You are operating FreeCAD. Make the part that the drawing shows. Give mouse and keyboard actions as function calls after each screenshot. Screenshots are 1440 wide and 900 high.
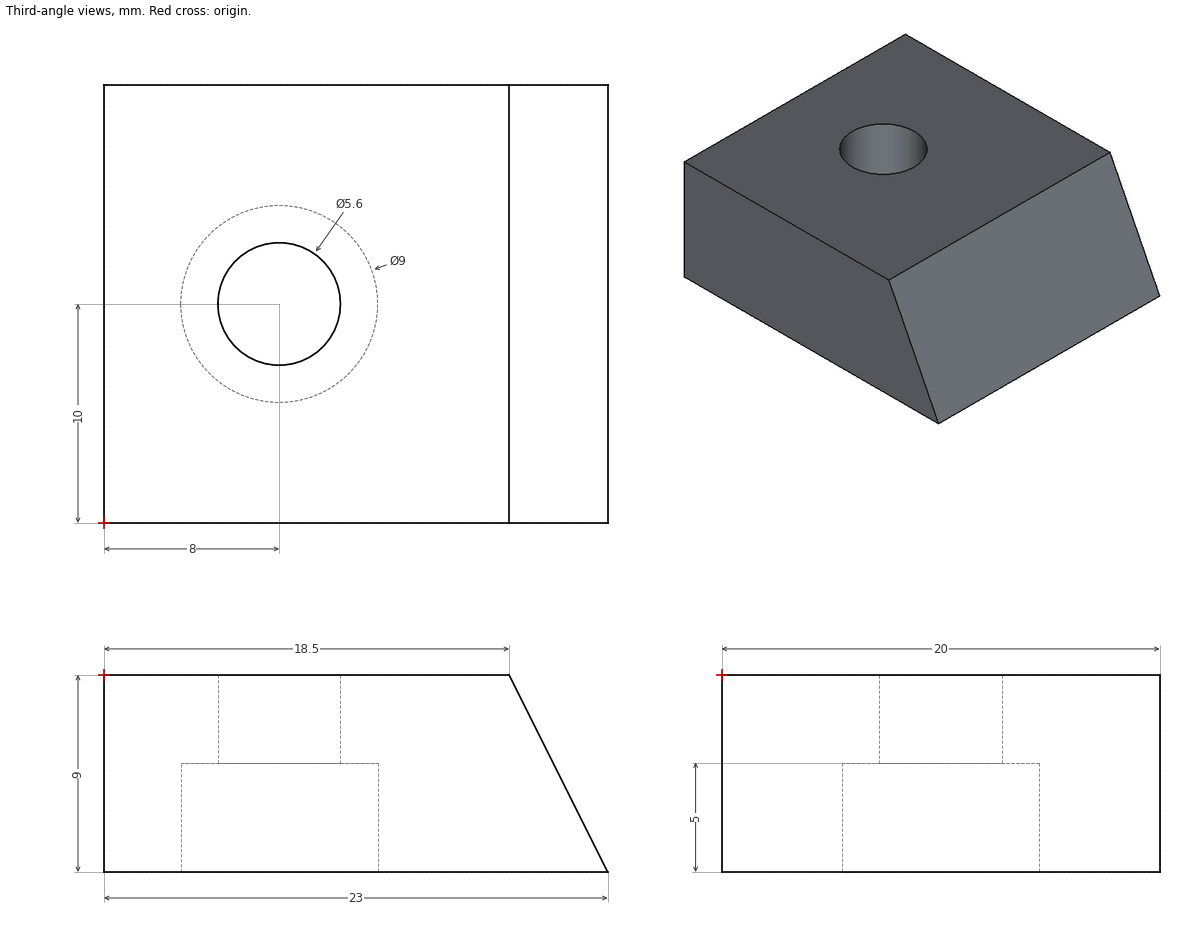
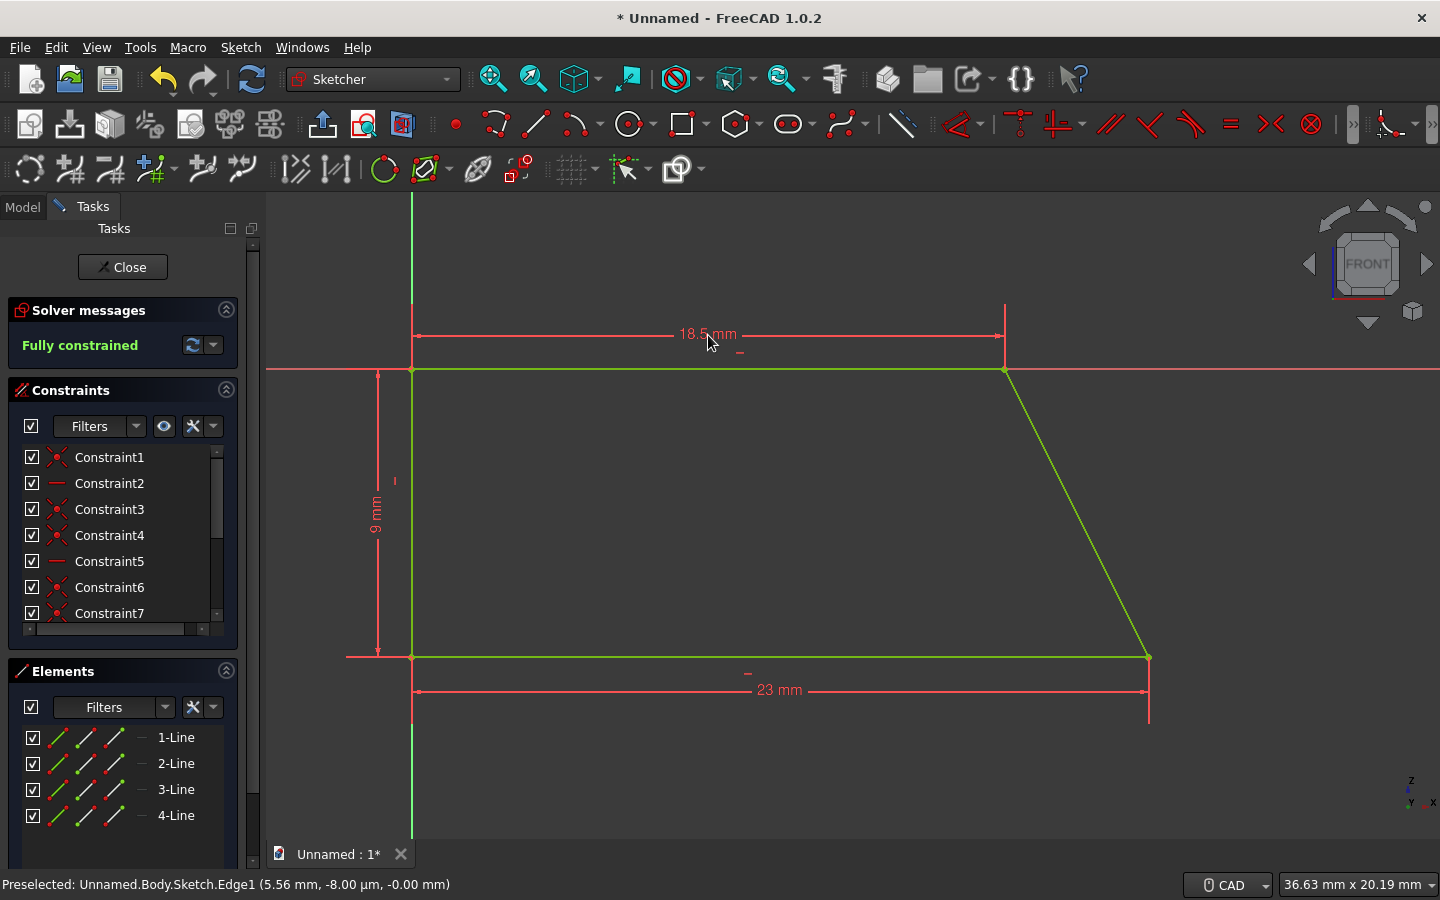
click(123, 267)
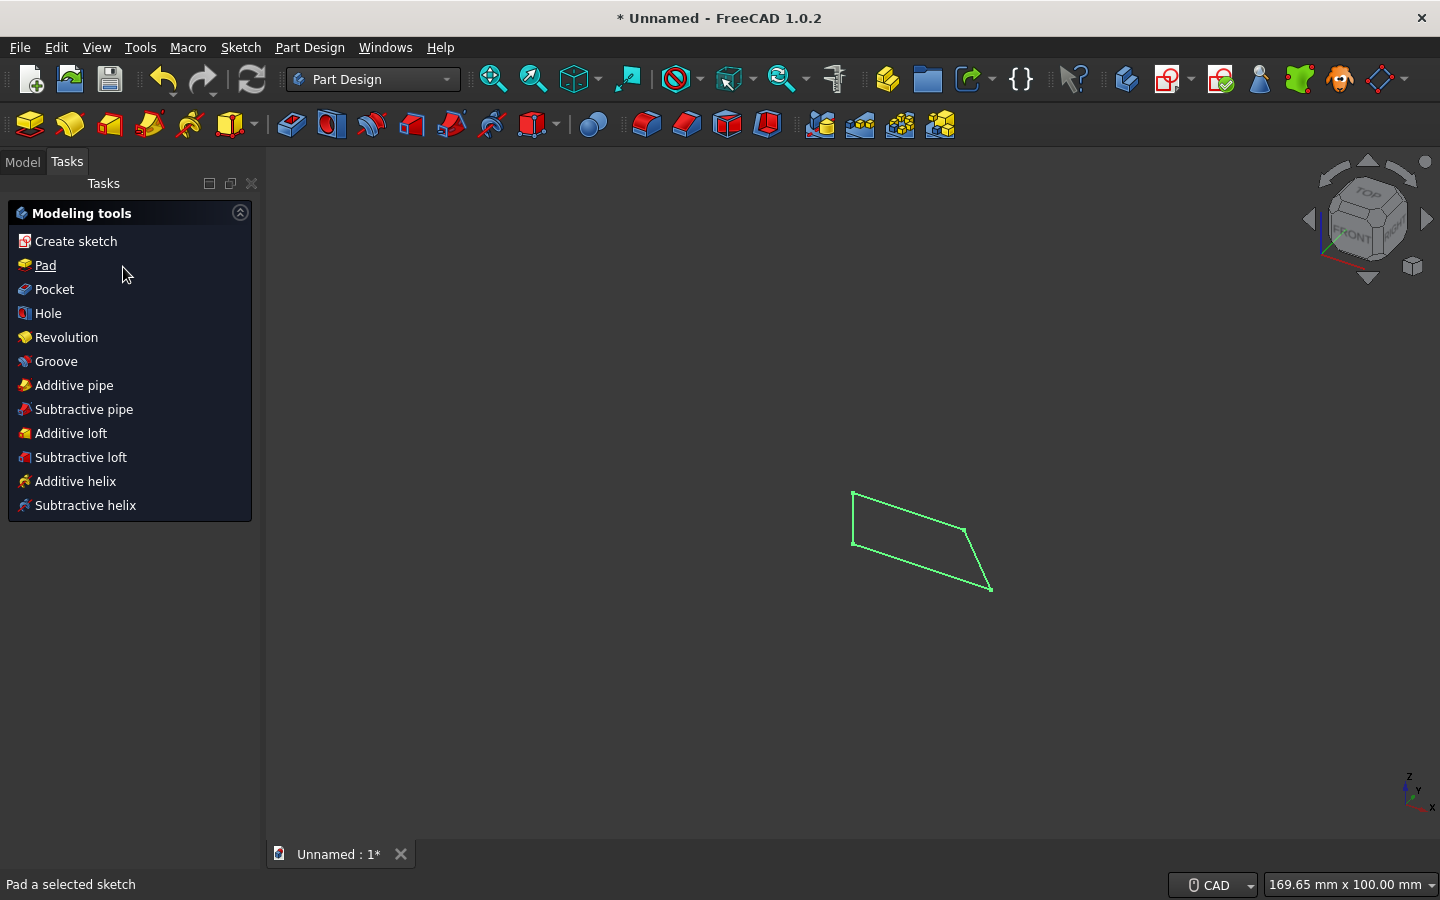
click(30, 124)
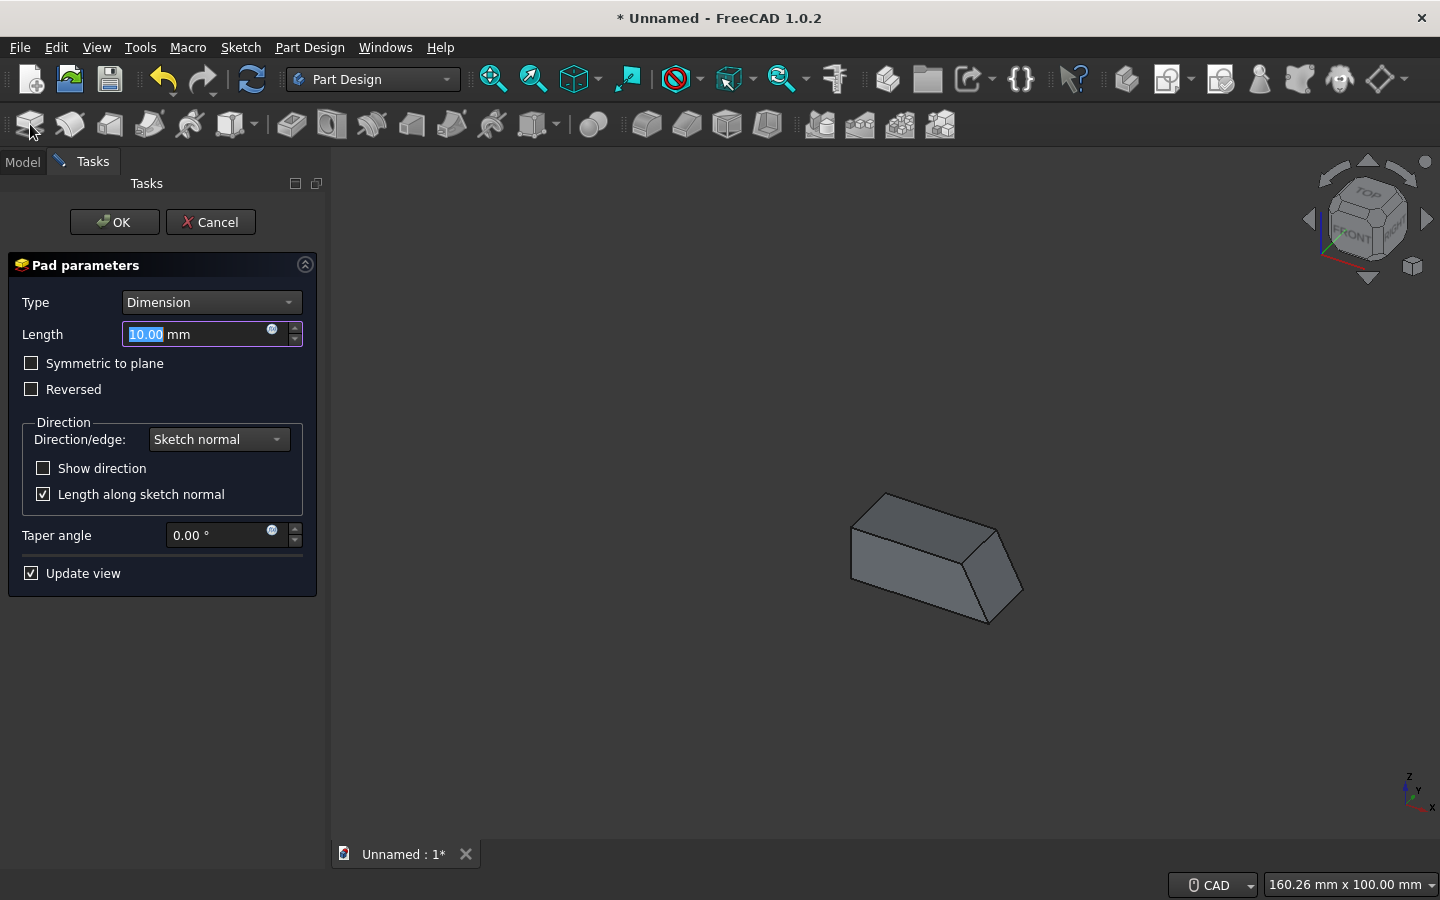
text(20)
key(Tab)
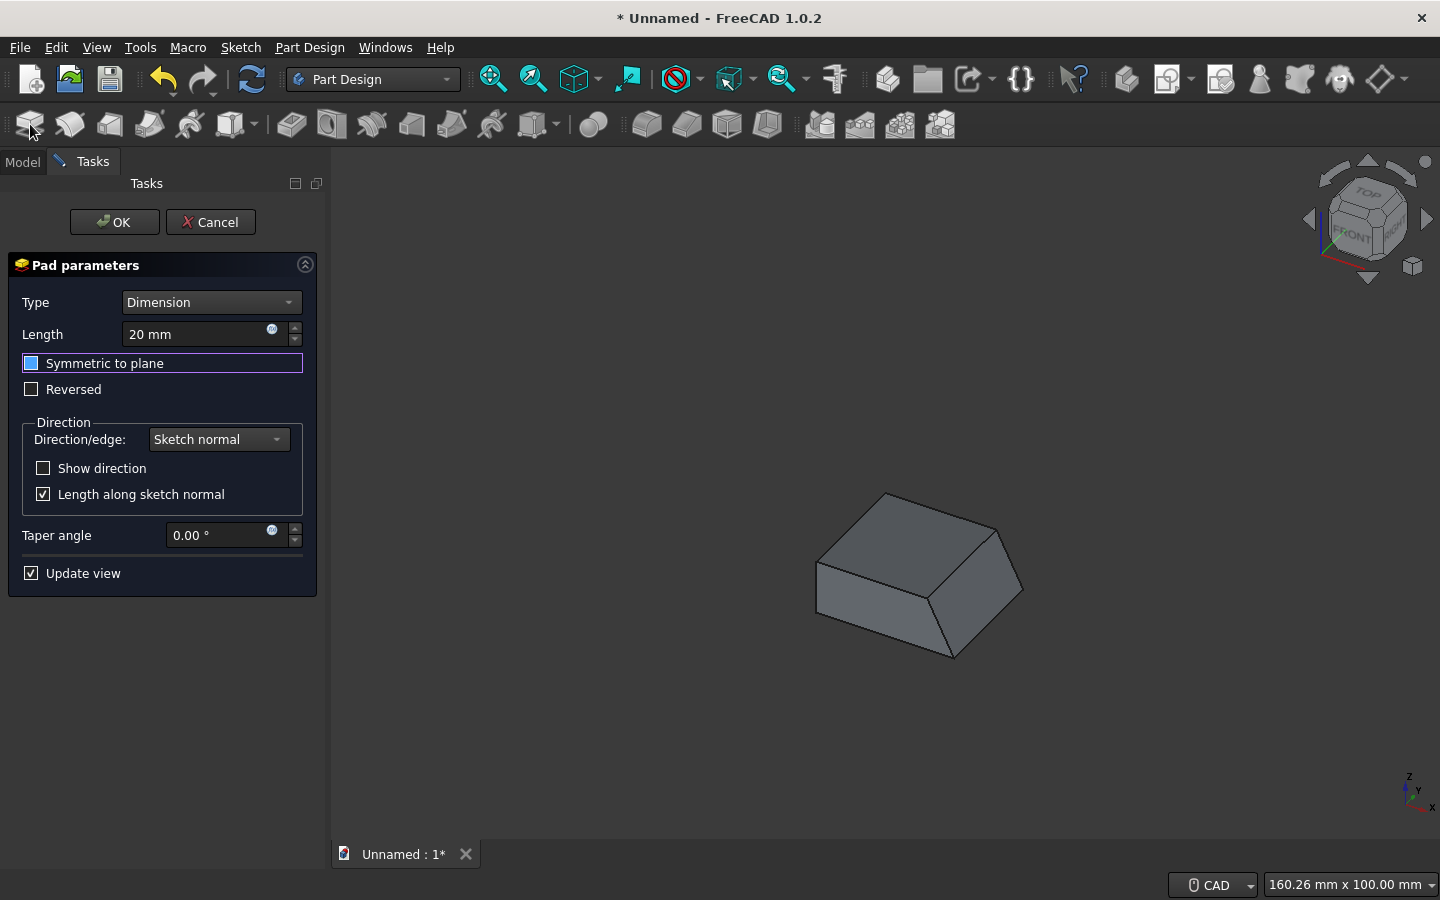
click(30, 389)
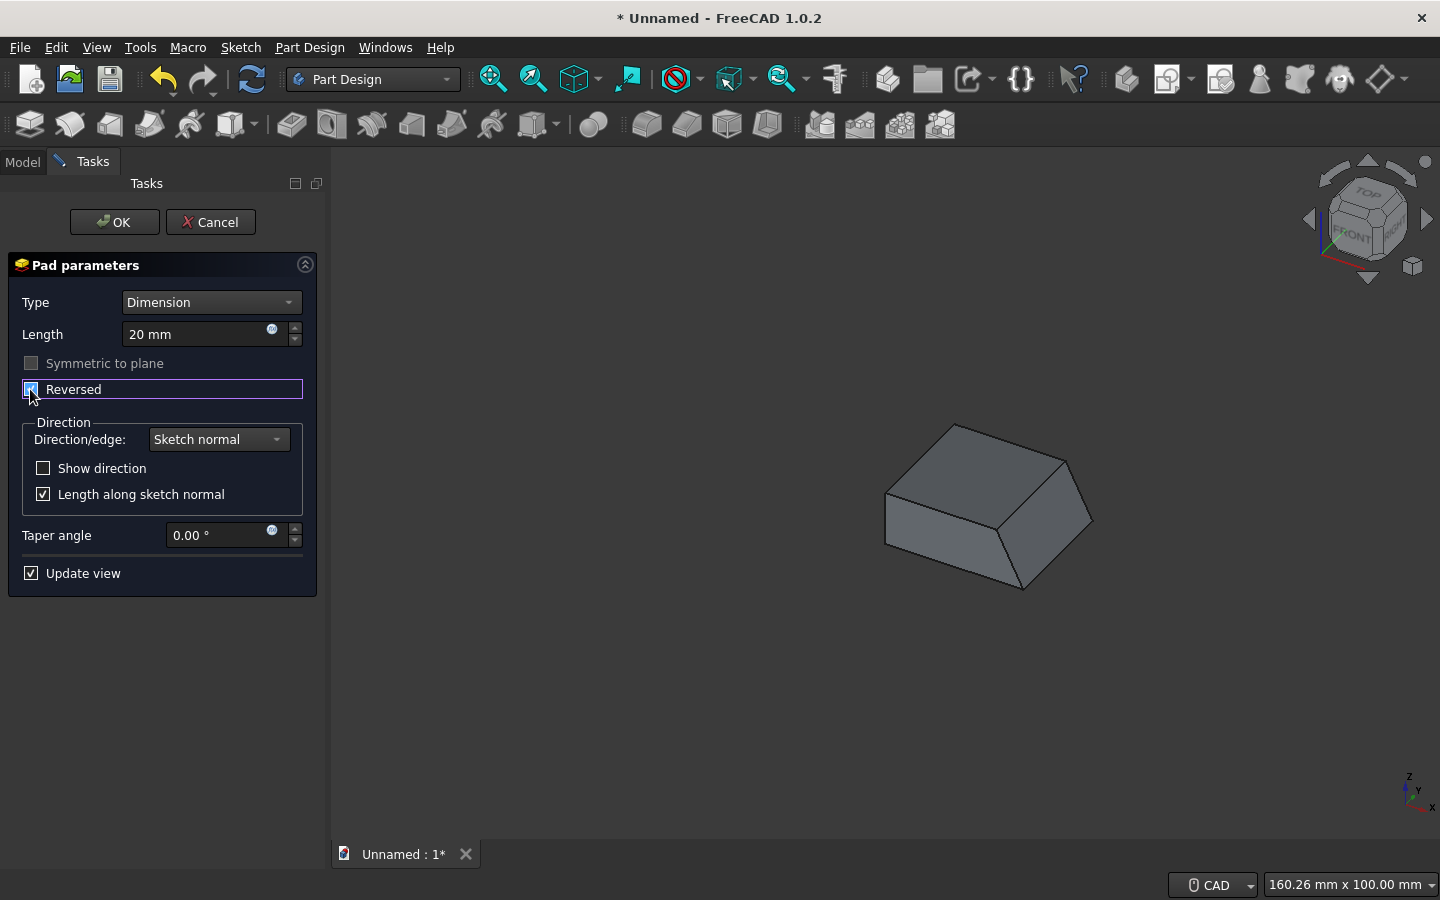
click(115, 222)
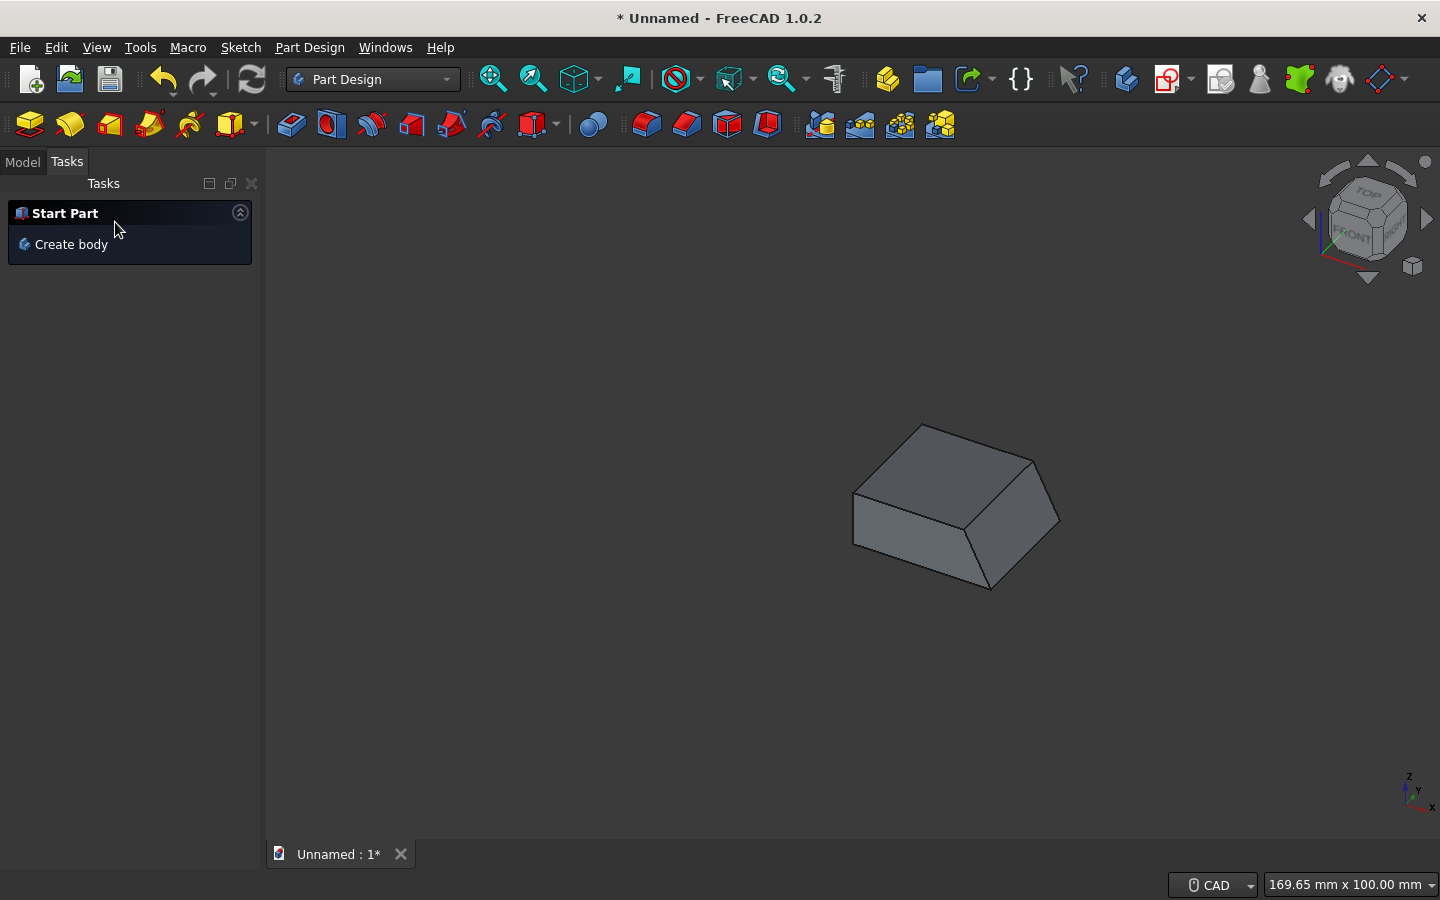
key(v)
key(f)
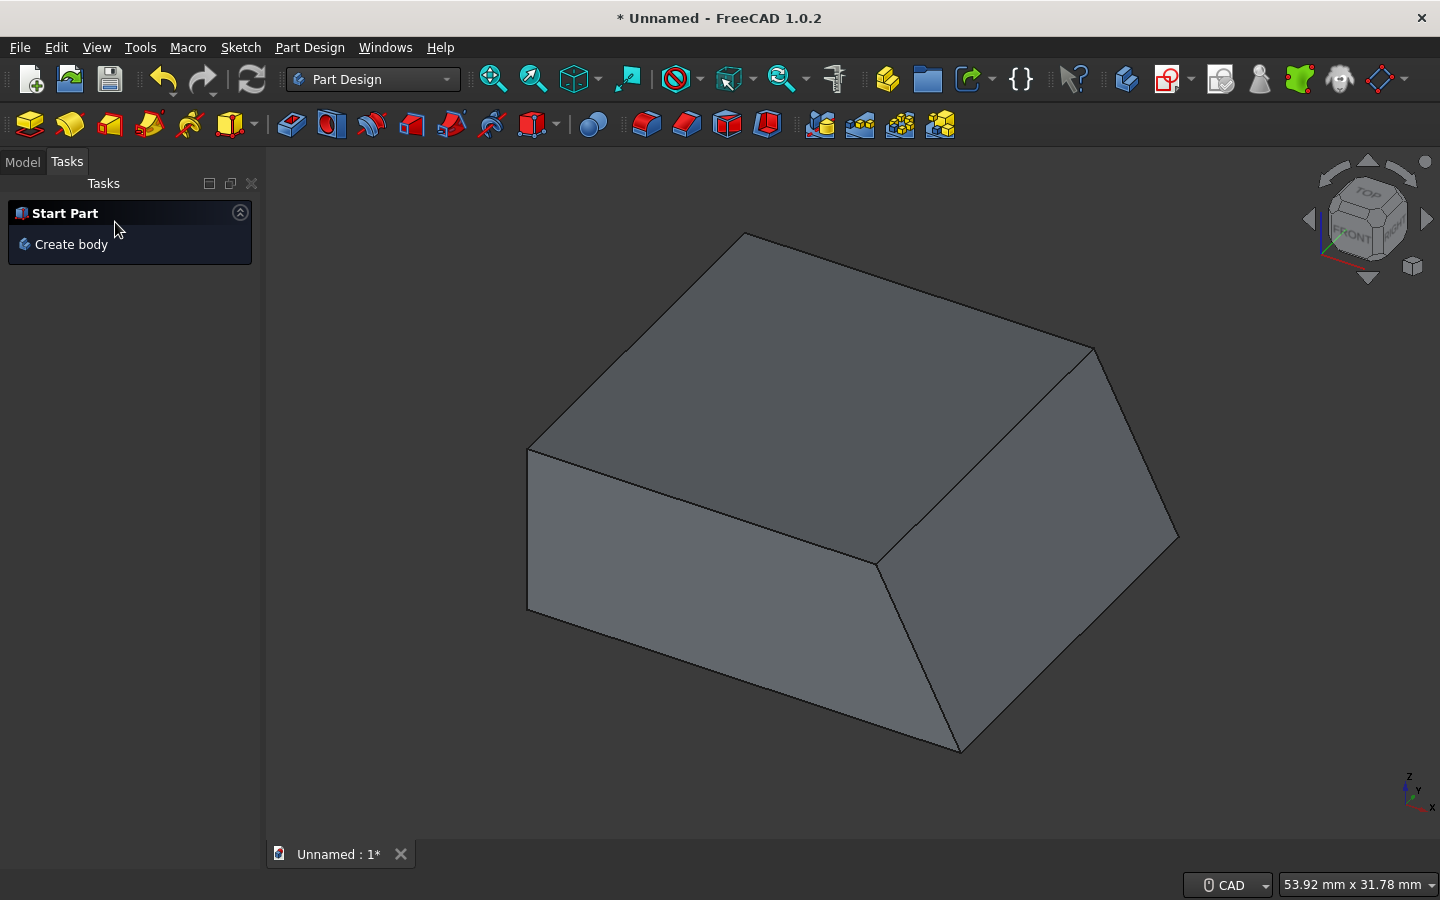
key(5)